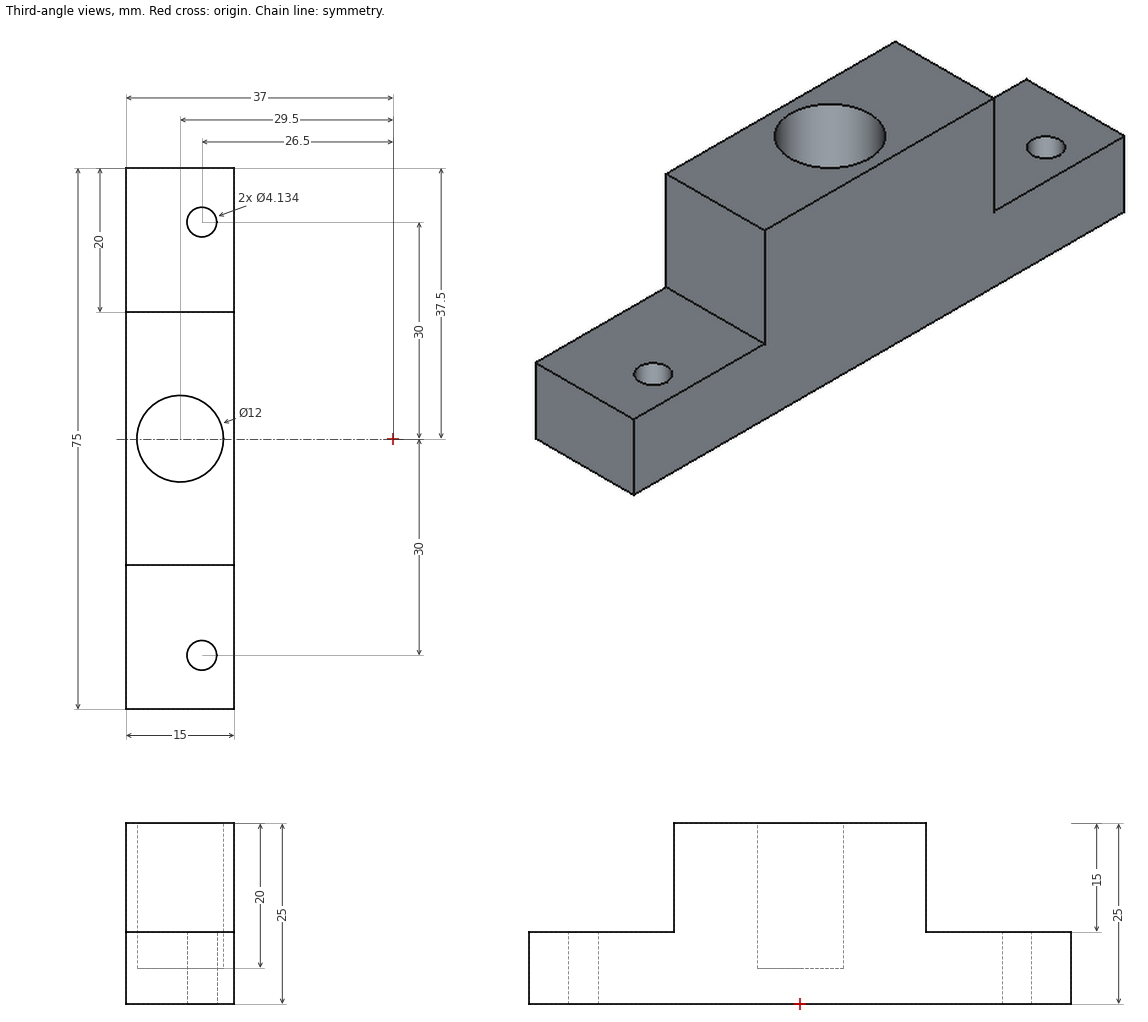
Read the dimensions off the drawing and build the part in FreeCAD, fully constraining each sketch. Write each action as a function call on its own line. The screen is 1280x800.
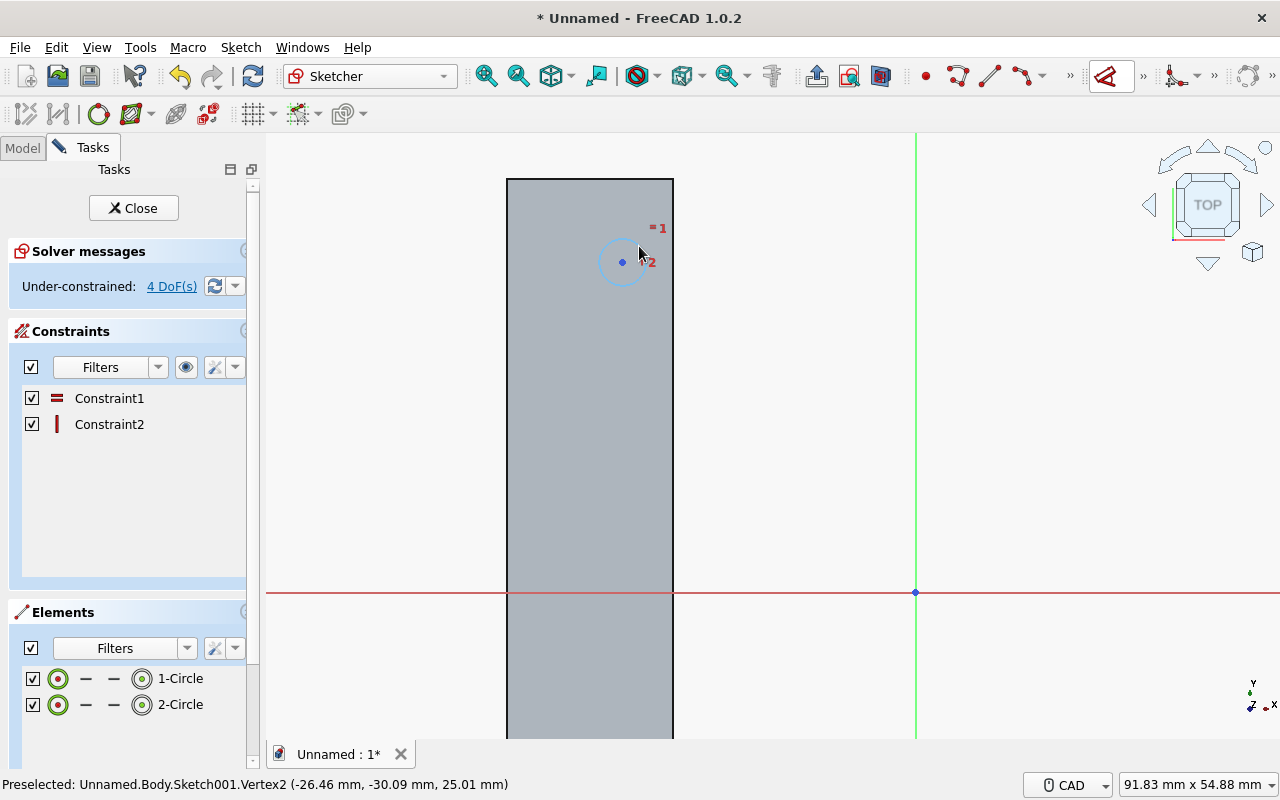
click(639, 246)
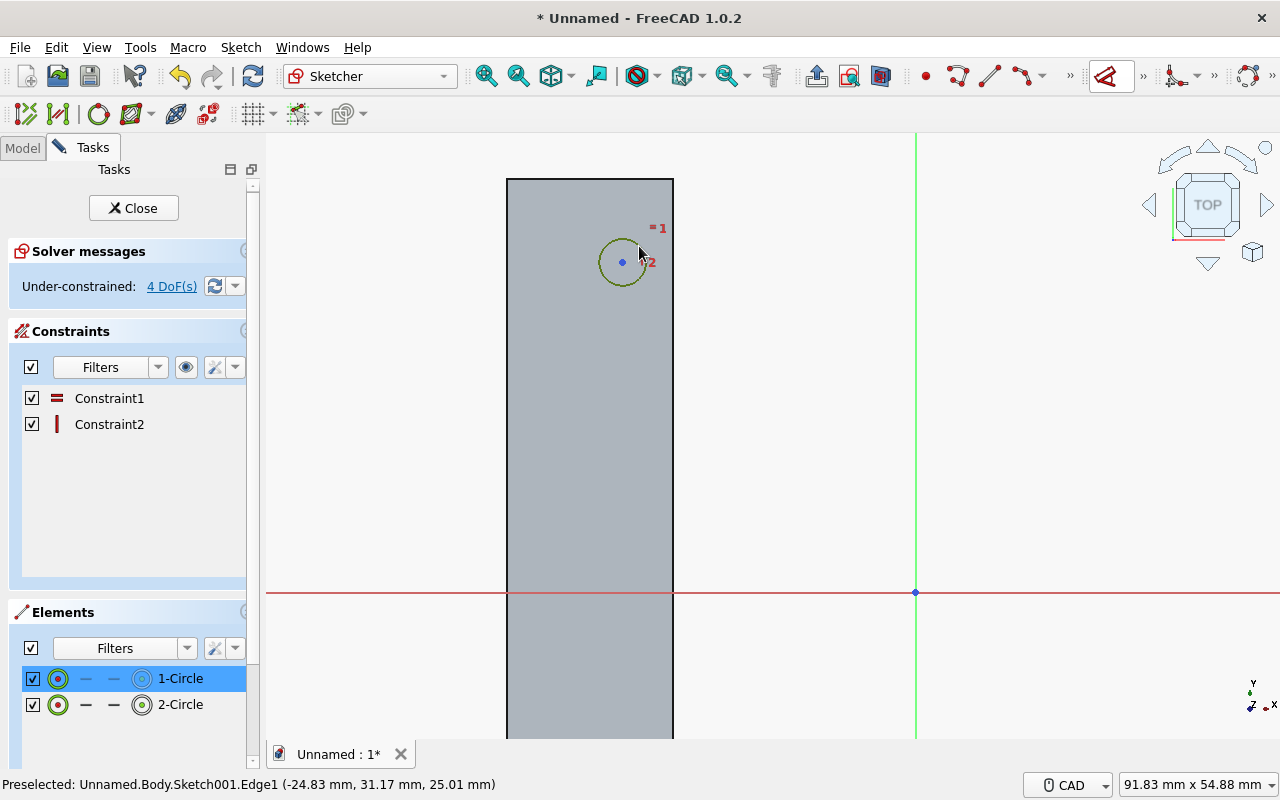
click(1128, 76)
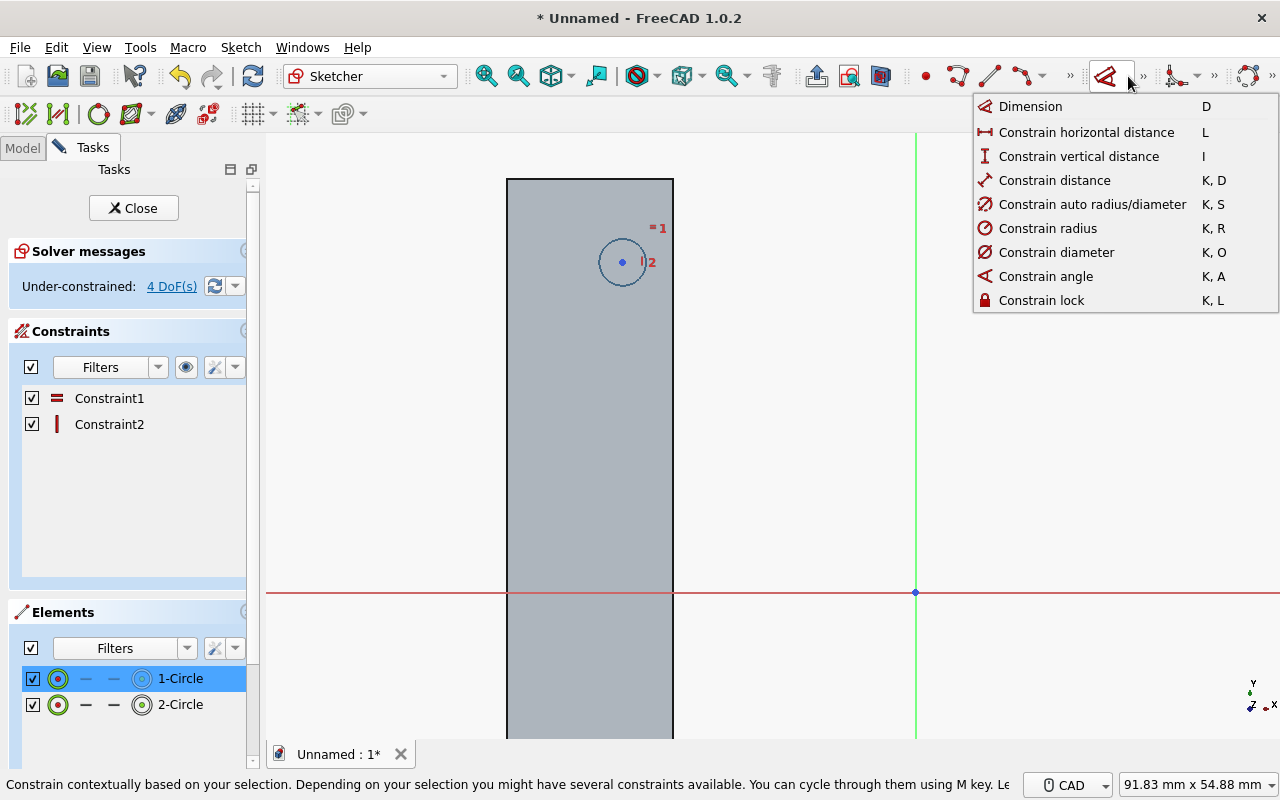
click(1126, 252)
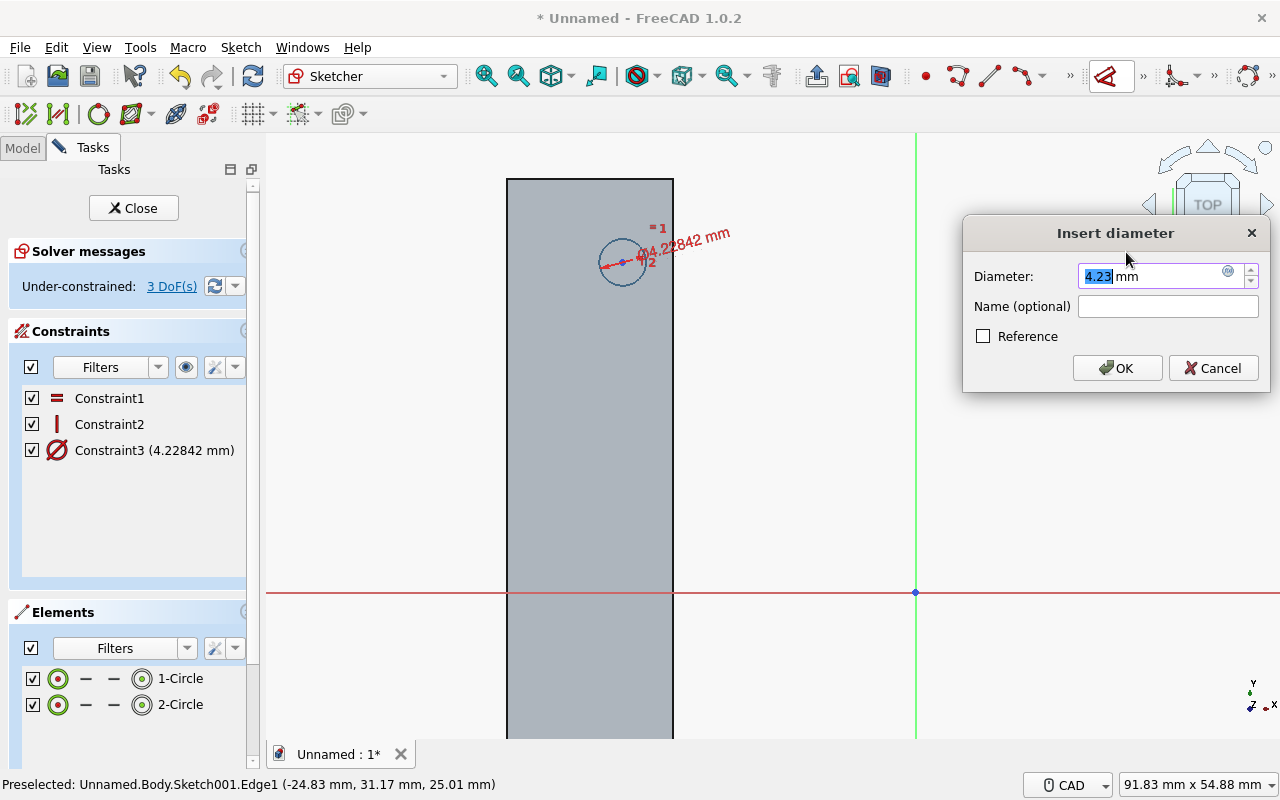
text(4.134)
key(Return)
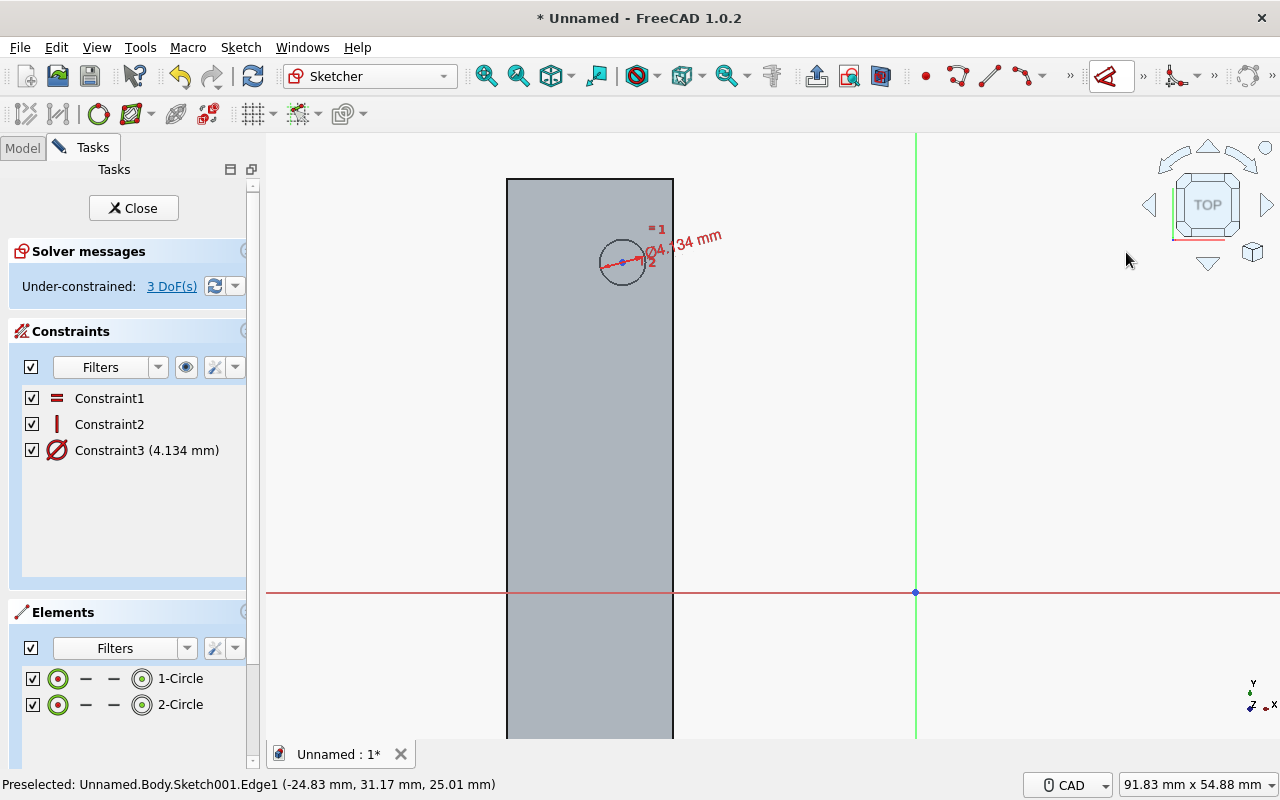
click(623, 262)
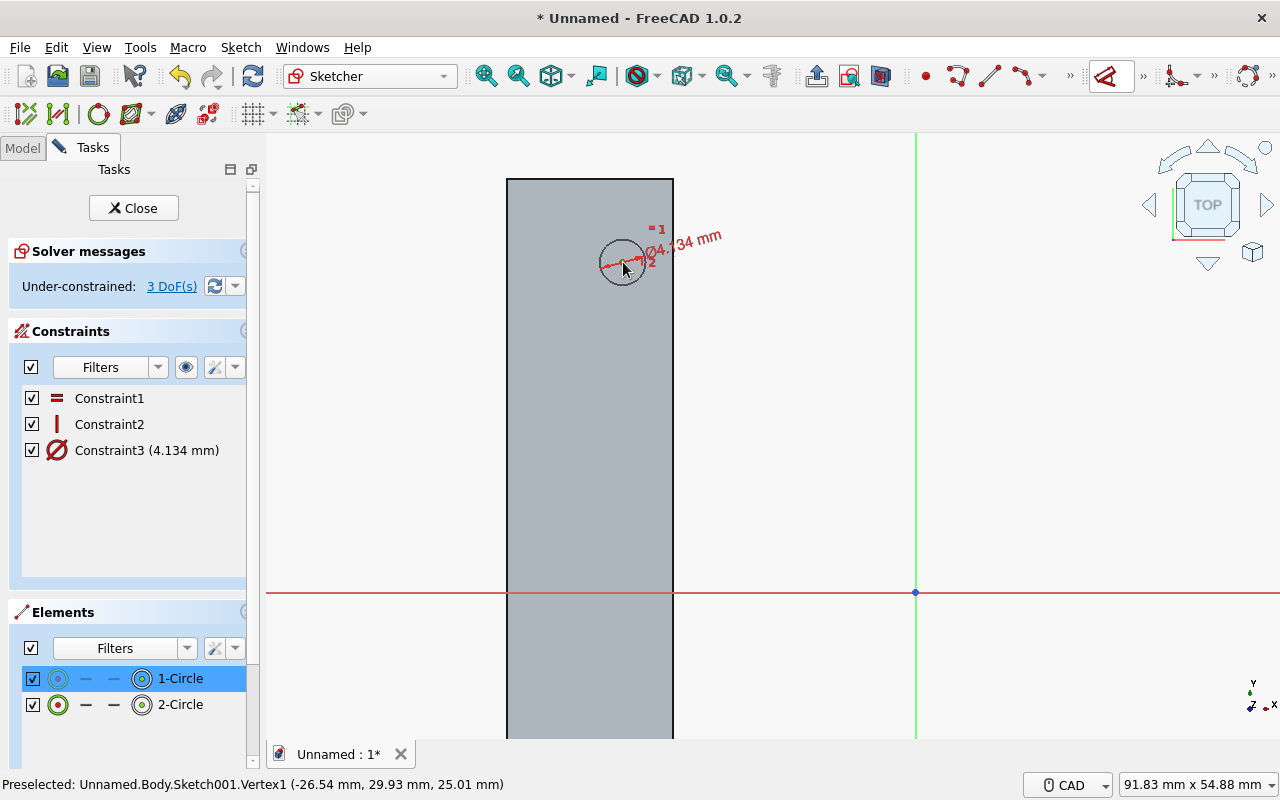
click(1128, 76)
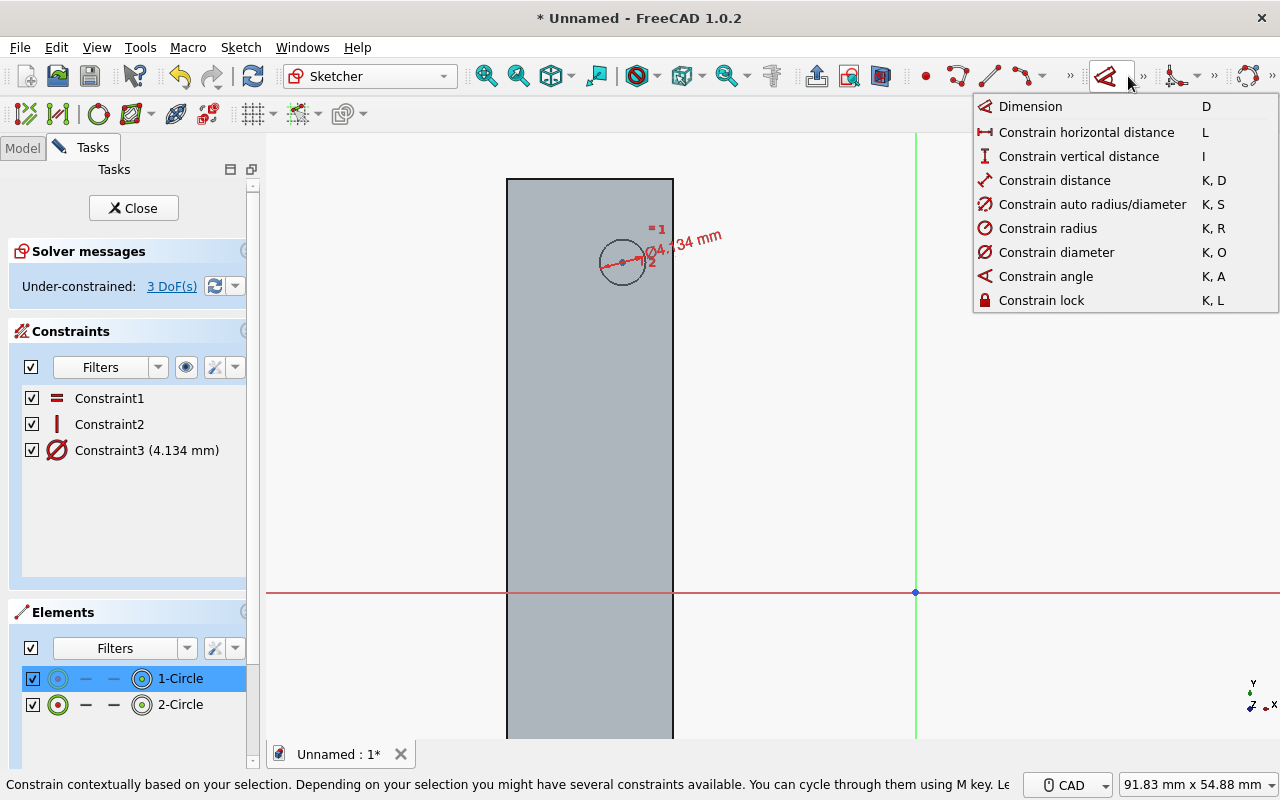
click(1126, 156)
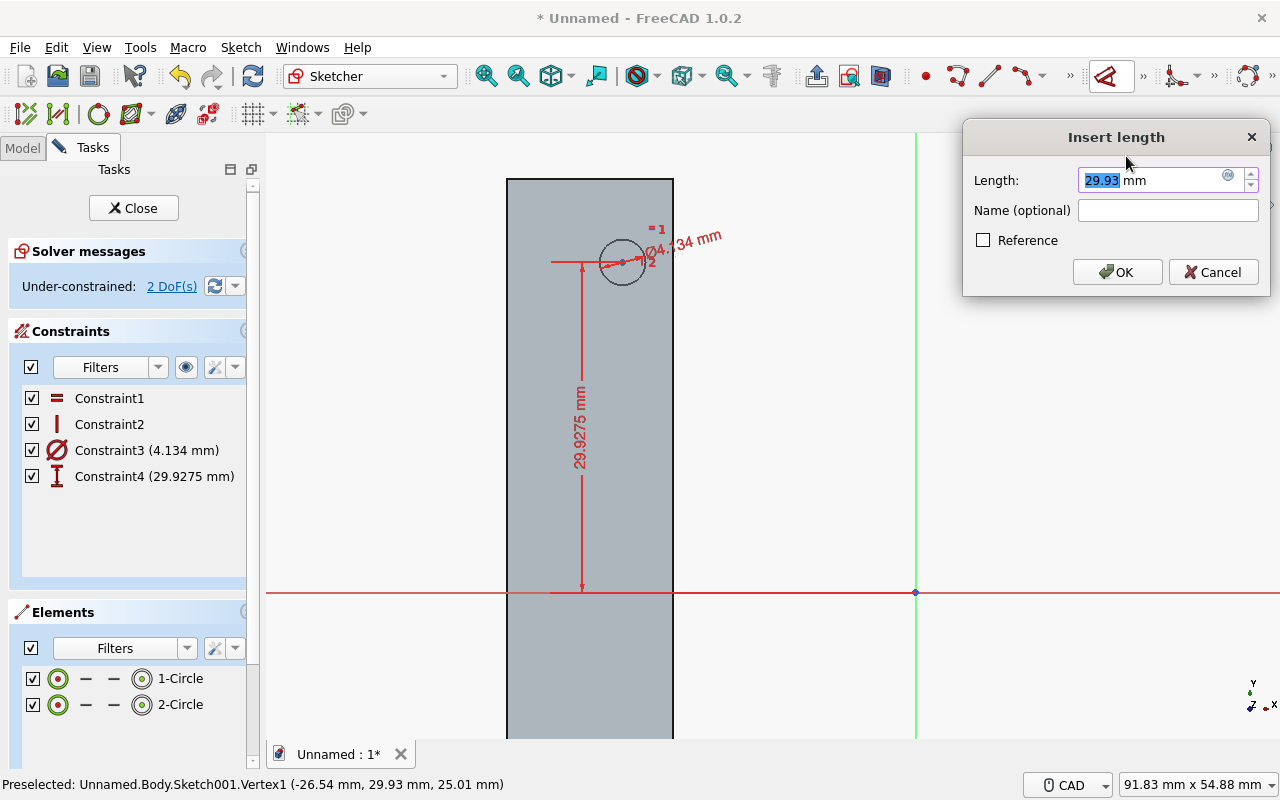
text(30)
key(Return)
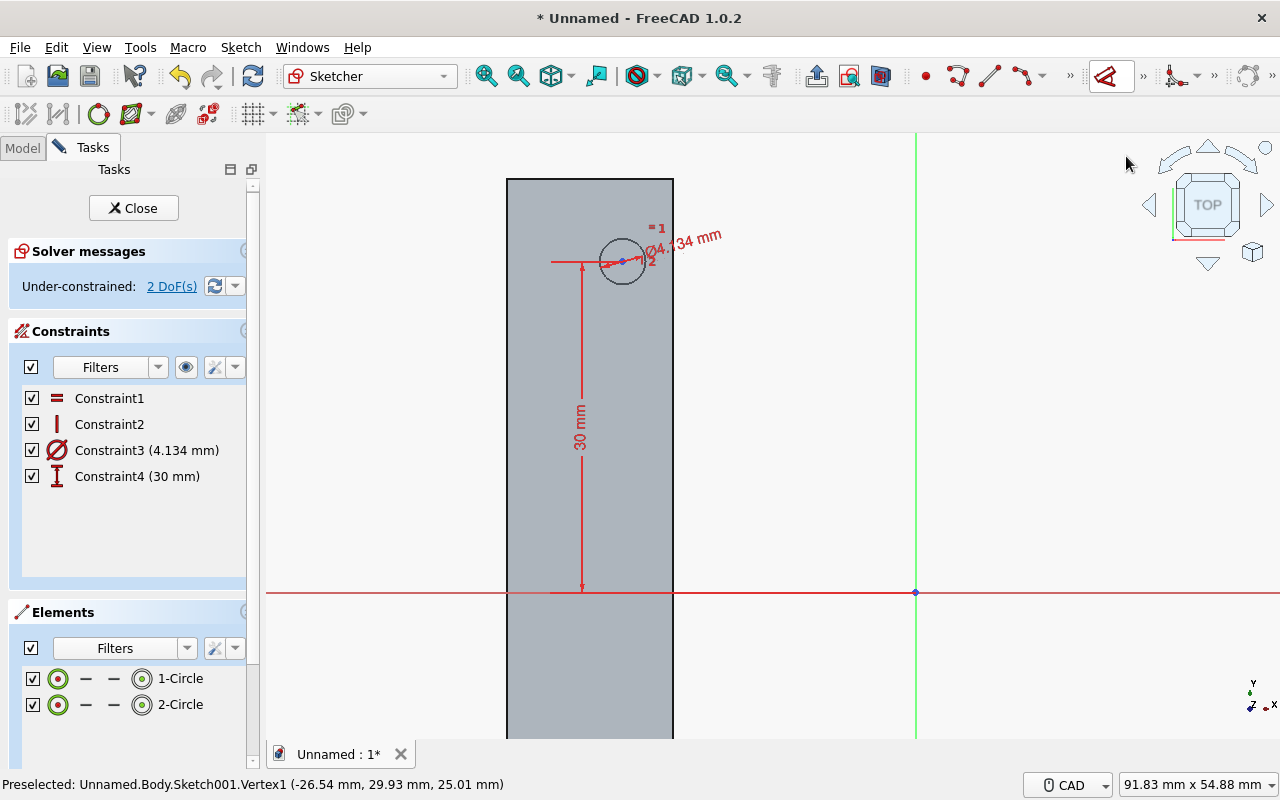
scroll(639, 245, down, 3)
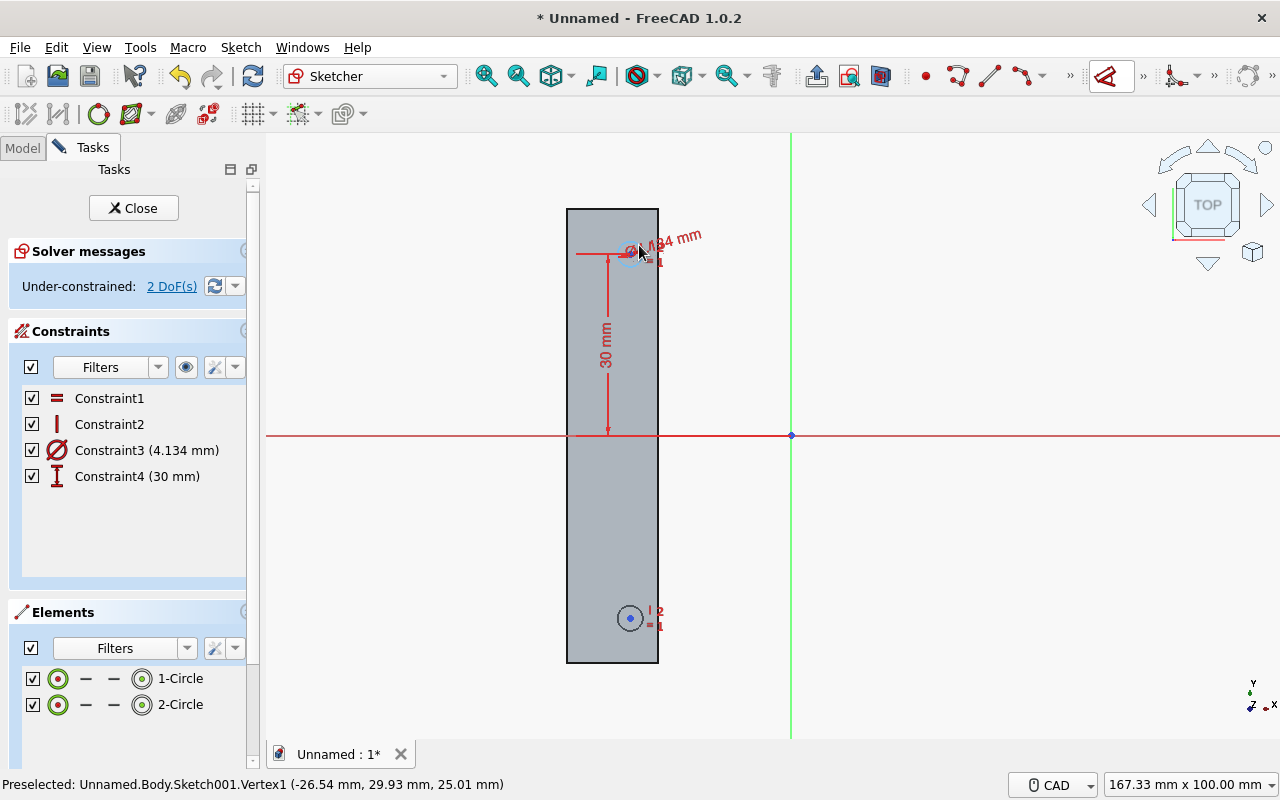
click(630, 618)